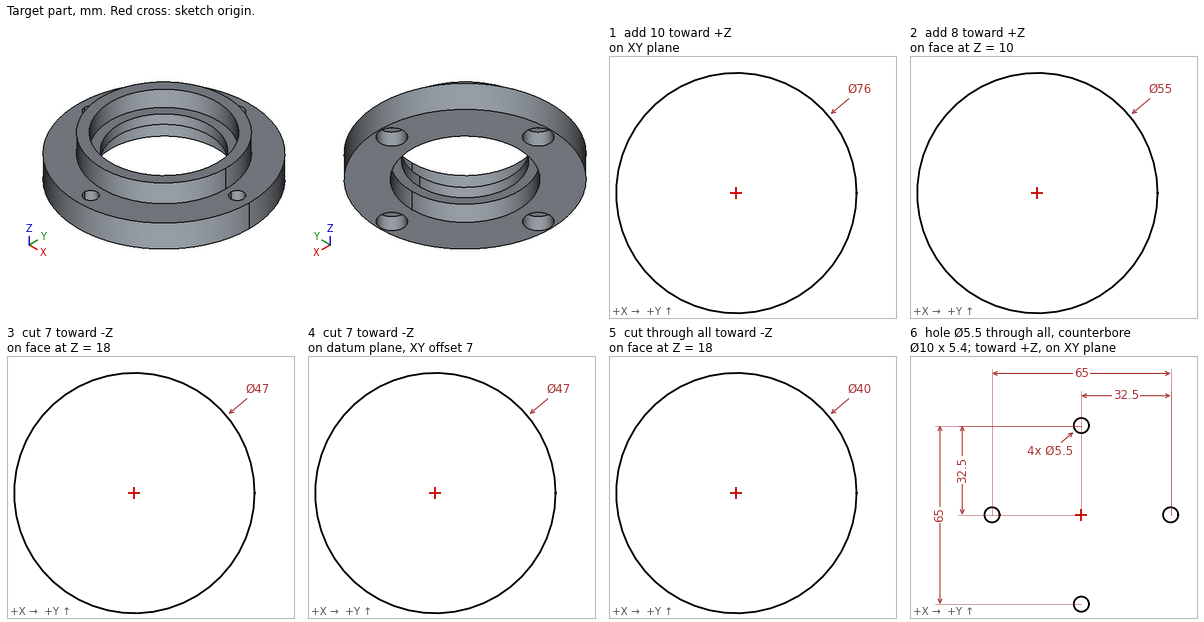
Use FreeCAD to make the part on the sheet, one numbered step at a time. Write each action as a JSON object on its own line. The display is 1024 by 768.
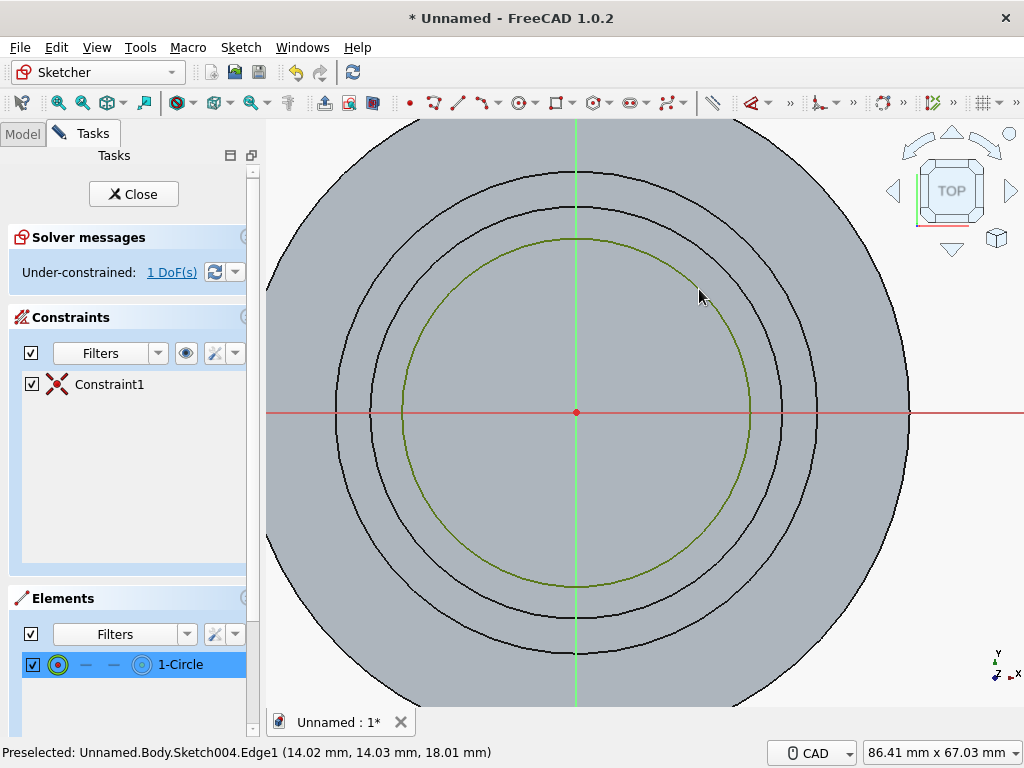
{"action": "left_click", "coordinate": [770, 104]}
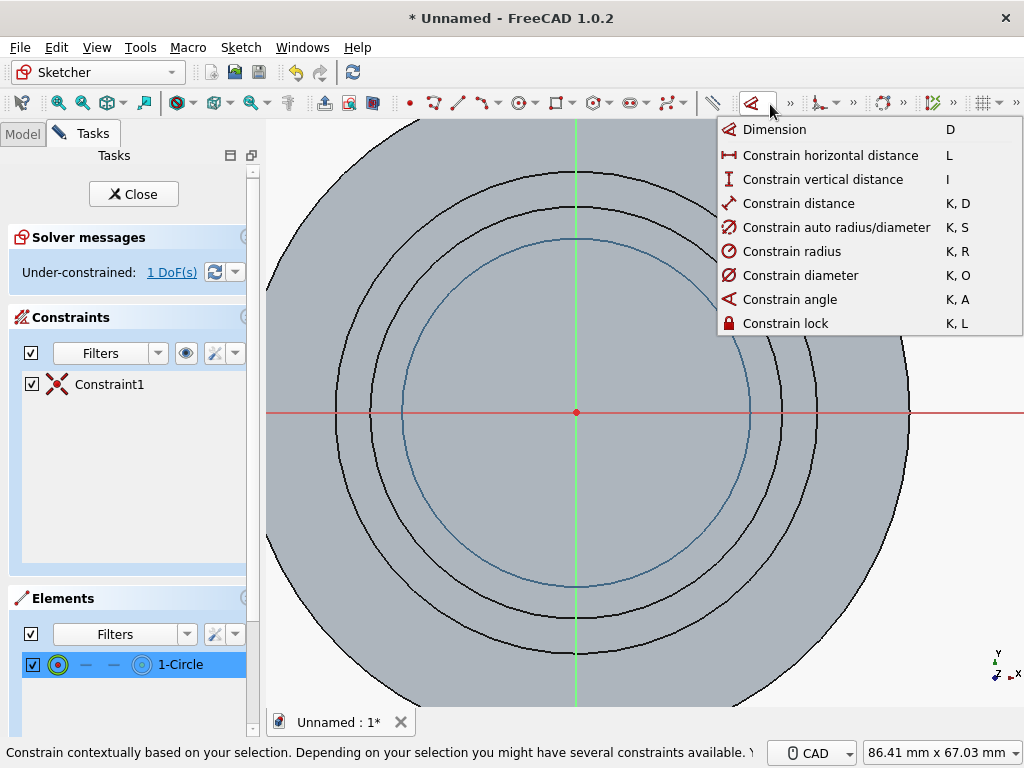
{"action": "left_click", "coordinate": [870, 275]}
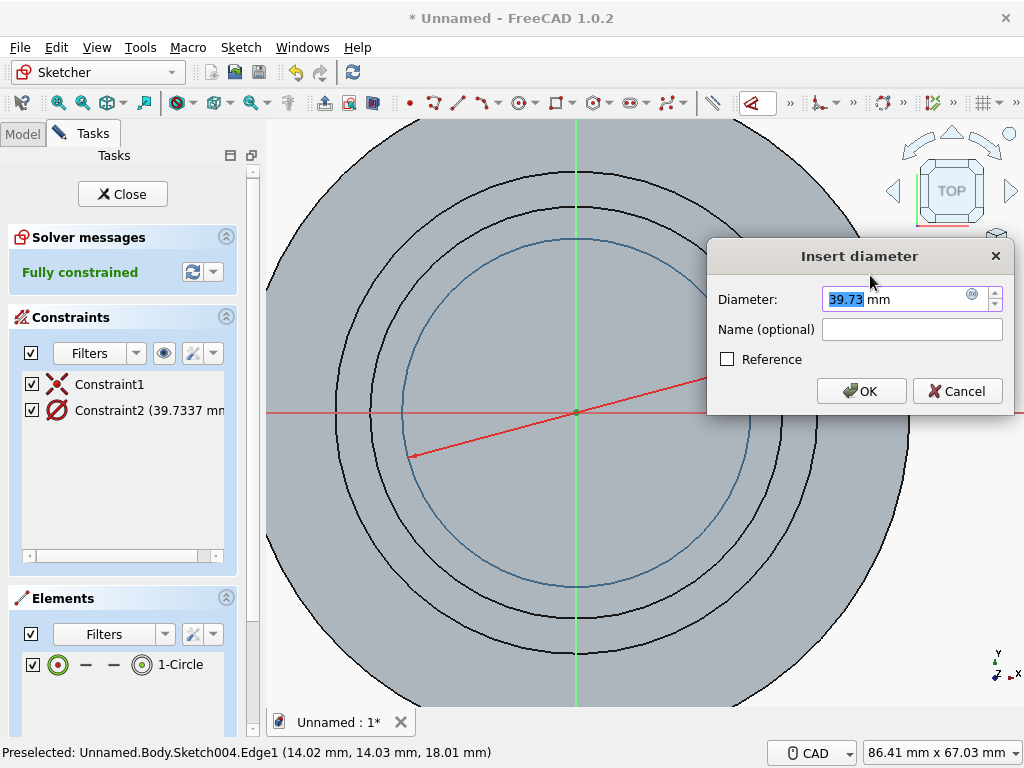
{"action": "type", "text": "40"}
{"action": "key", "text": "Return"}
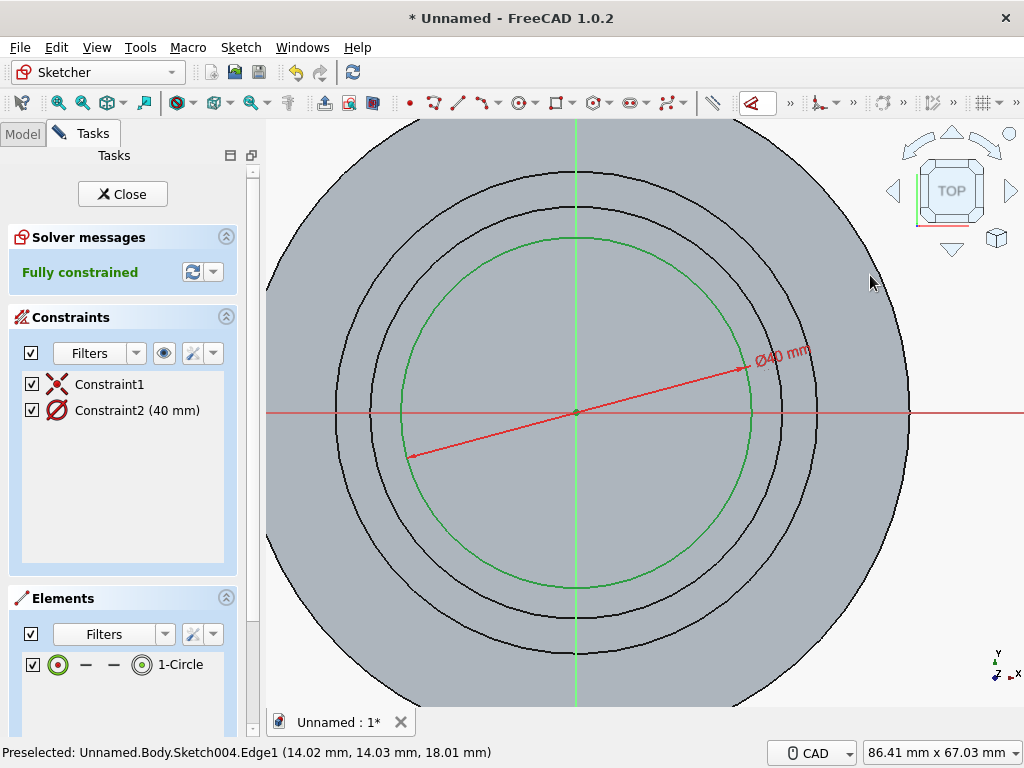
{"action": "left_click", "coordinate": [123, 194]}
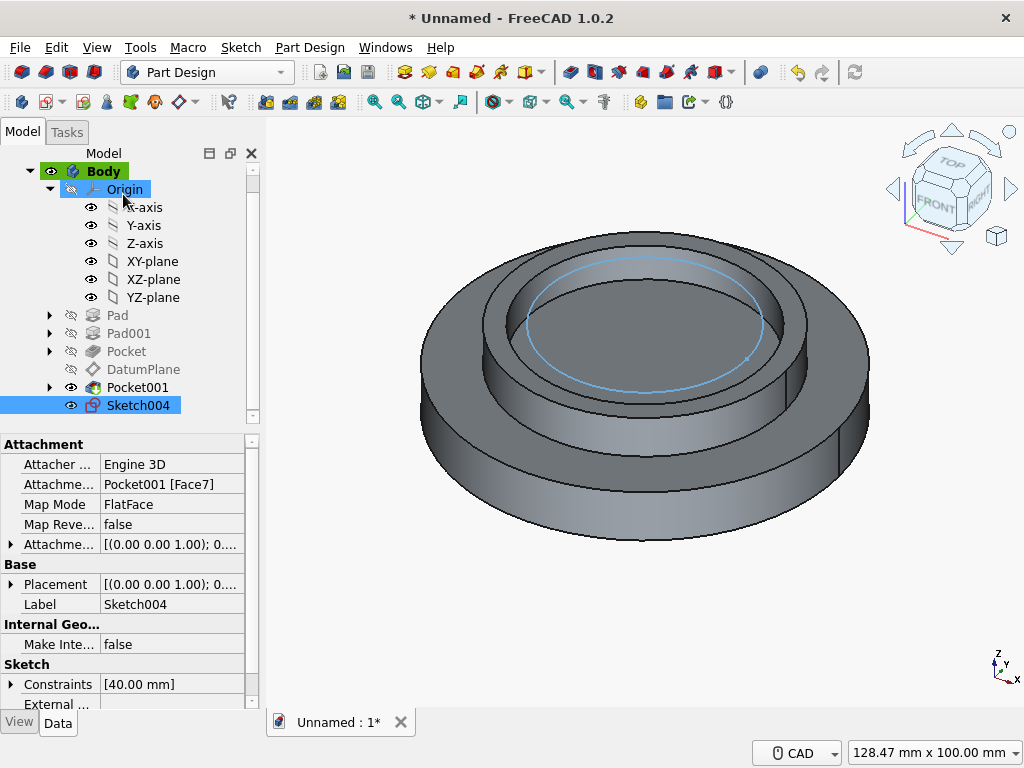
{"action": "left_click", "coordinate": [572, 72]}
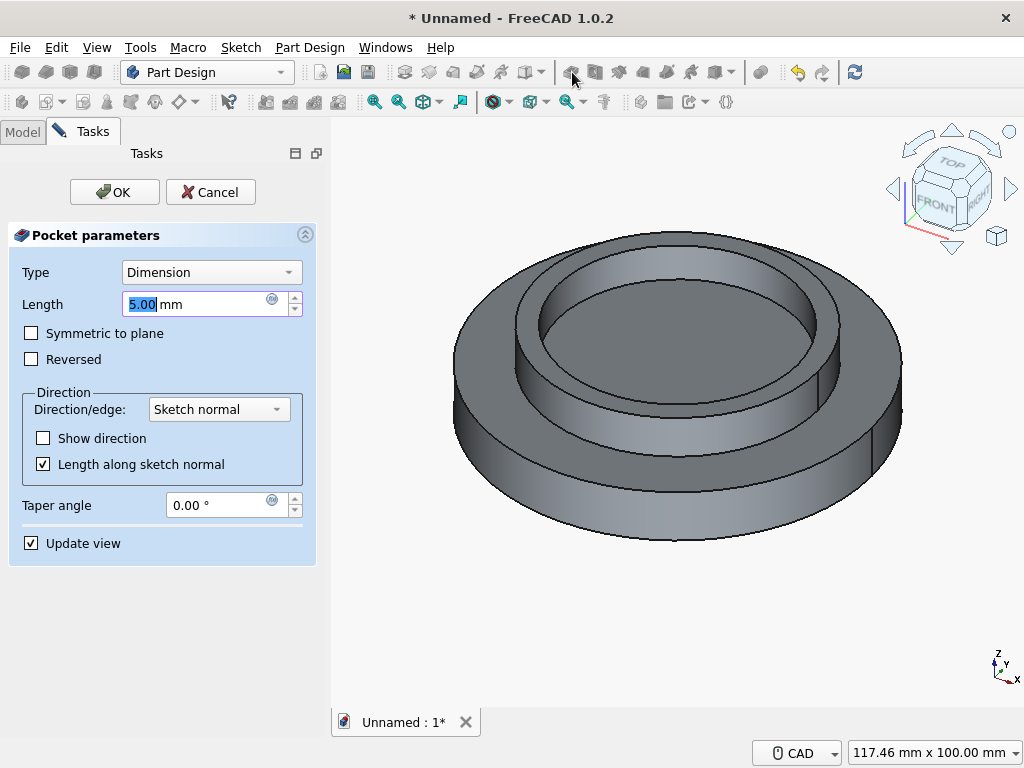
{"action": "left_click", "coordinate": [212, 272]}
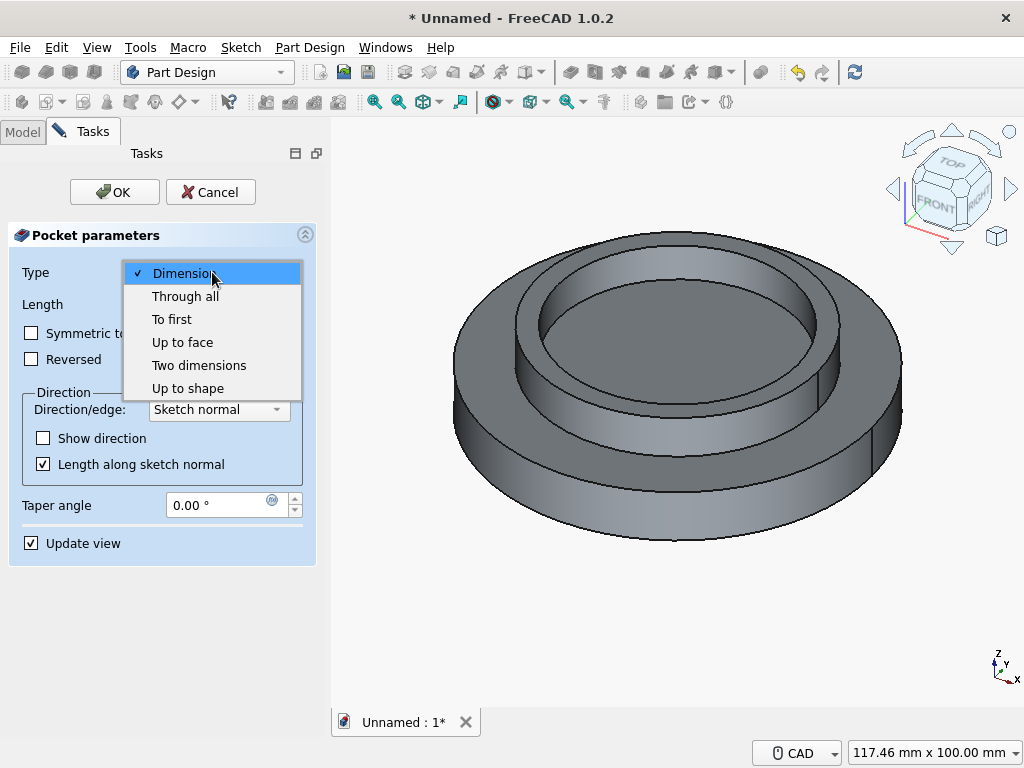
{"action": "left_click", "coordinate": [212, 296]}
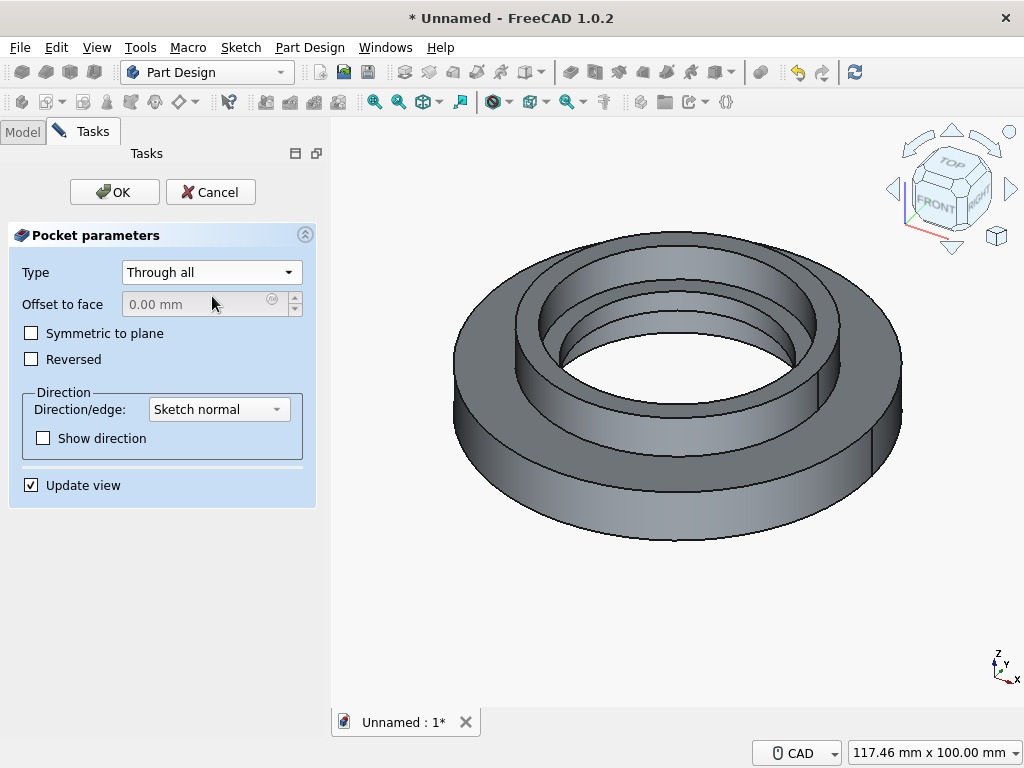
{"action": "left_click", "coordinate": [115, 192]}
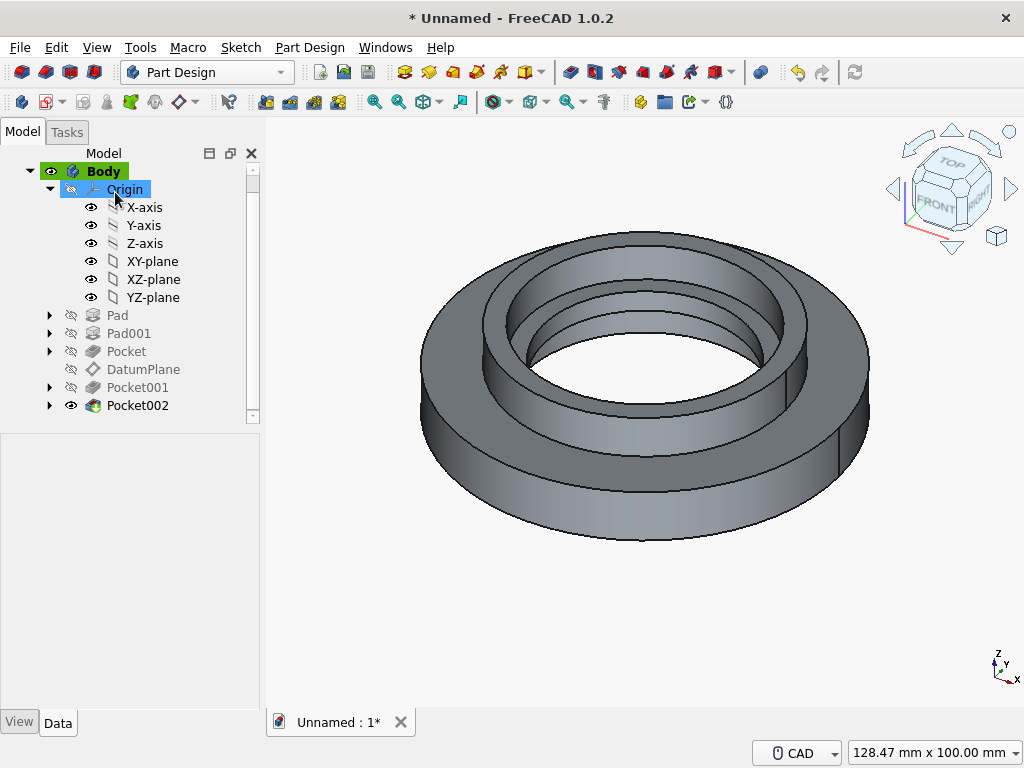
{"action": "left_click", "coordinate": [46, 102]}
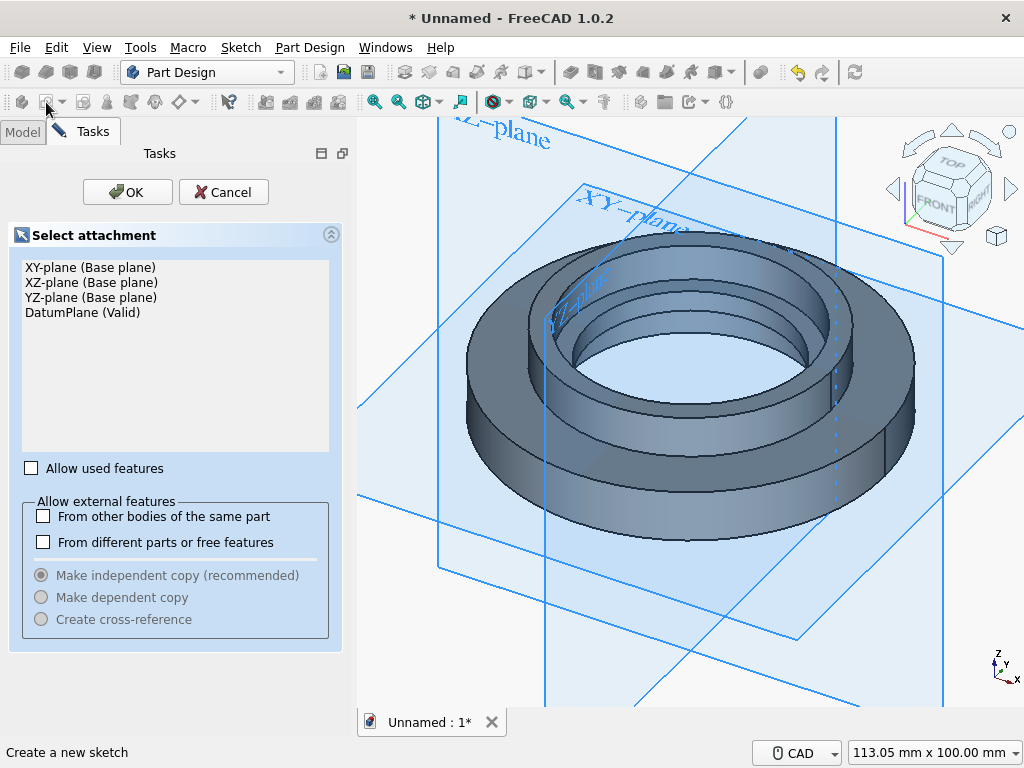
{"action": "left_click", "coordinate": [82, 268]}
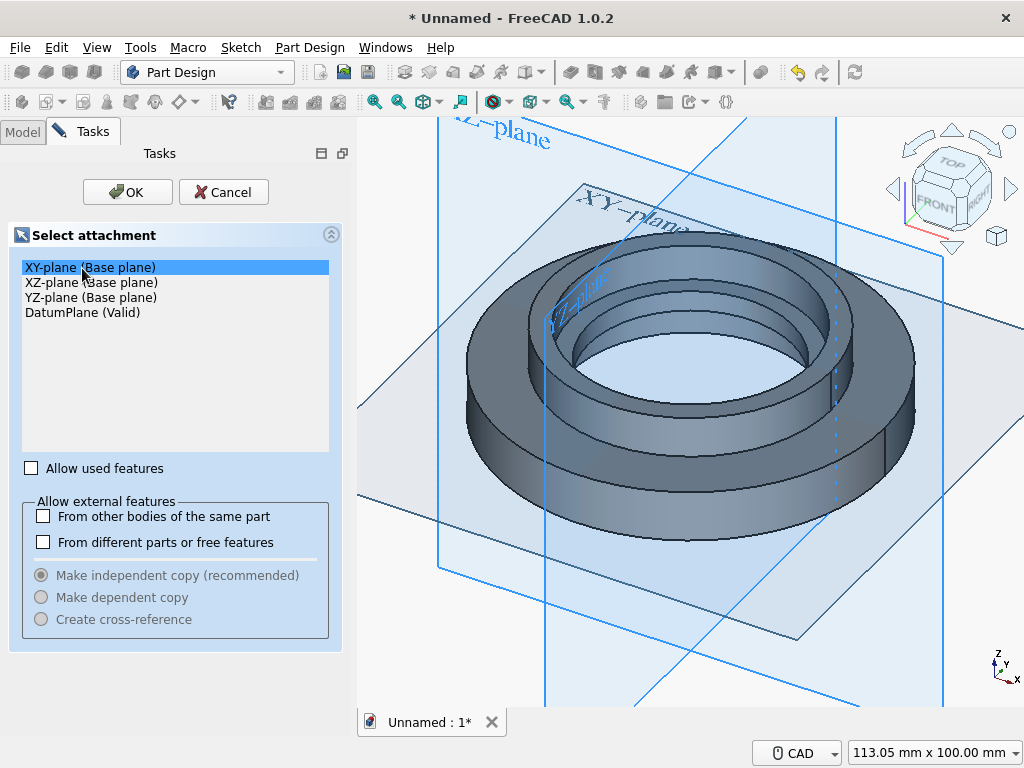
{"action": "left_click", "coordinate": [128, 192]}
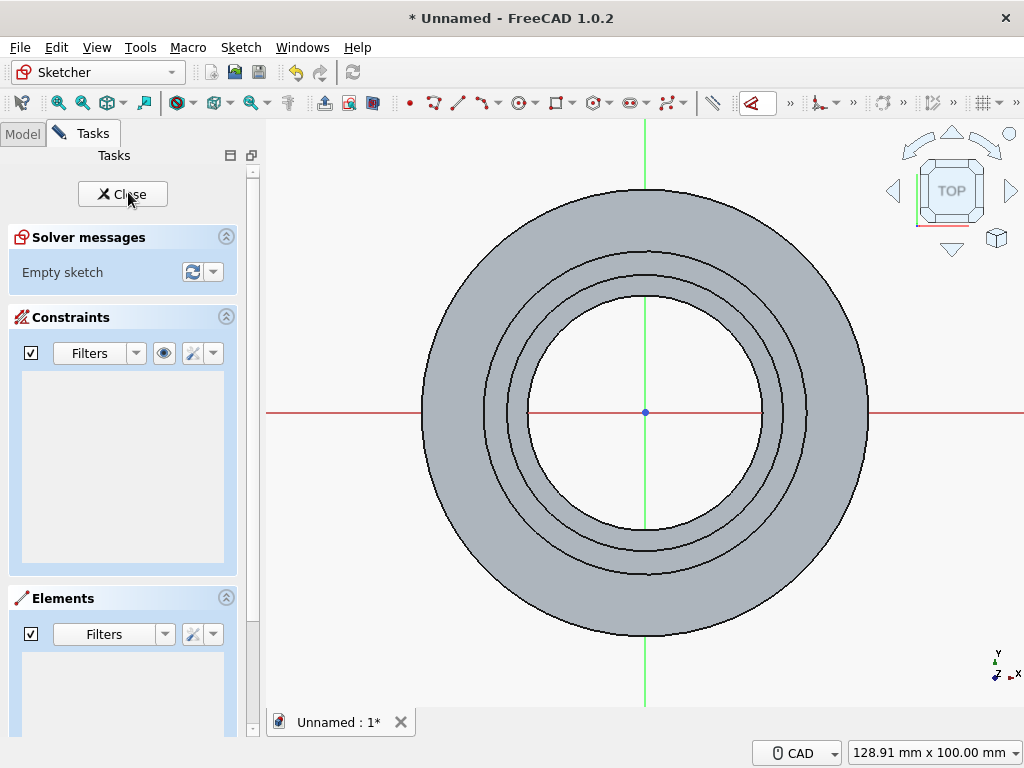
{"action": "key", "text": "q s"}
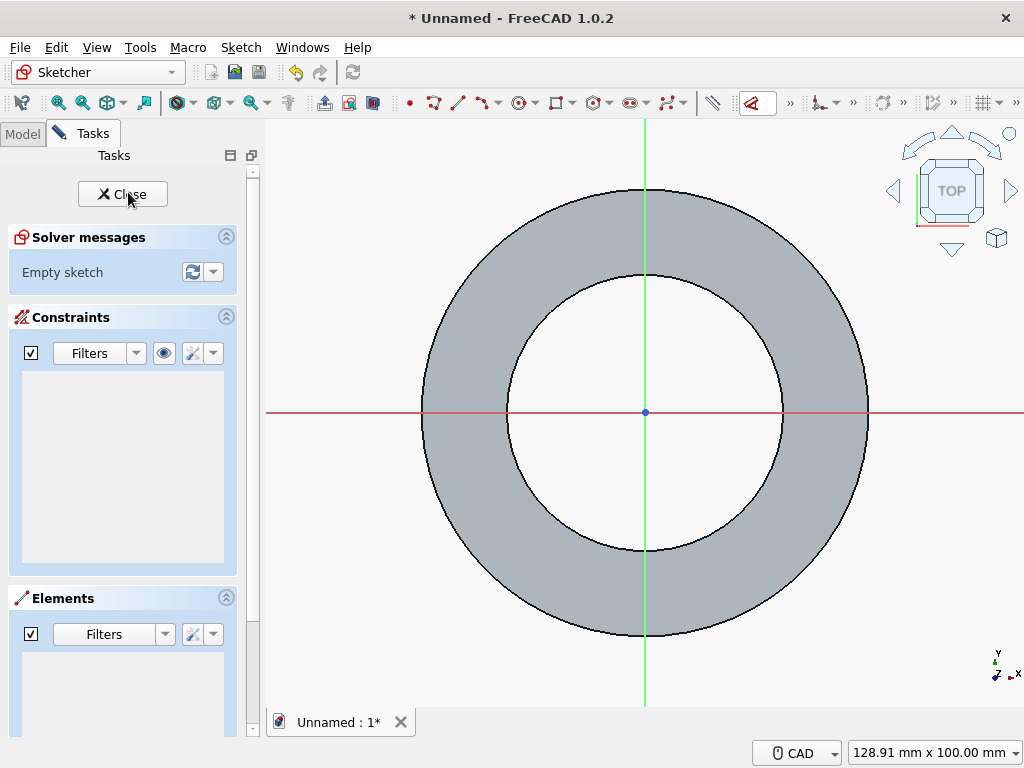
{"action": "scroll", "coordinate": [294, 413], "scroll_direction": "down", "scroll_amount": 1}